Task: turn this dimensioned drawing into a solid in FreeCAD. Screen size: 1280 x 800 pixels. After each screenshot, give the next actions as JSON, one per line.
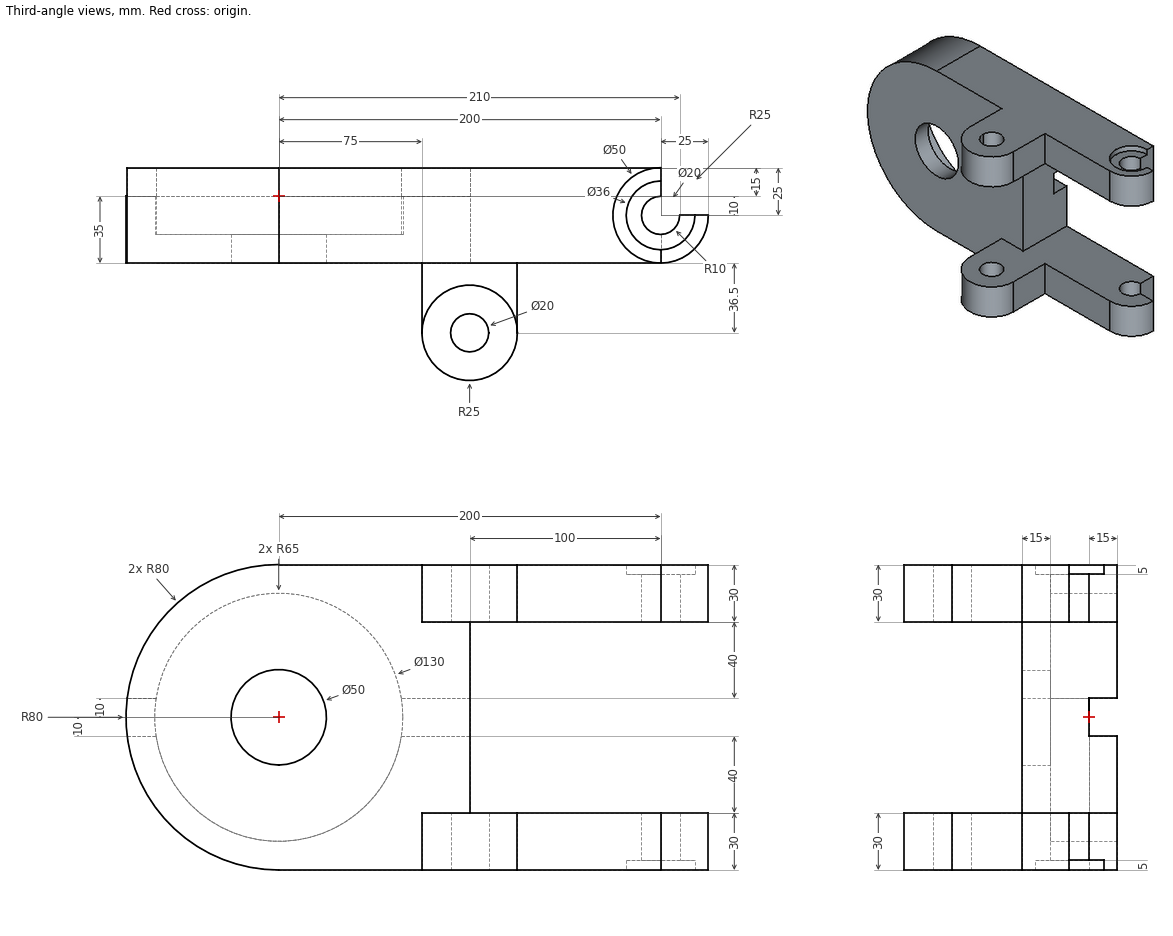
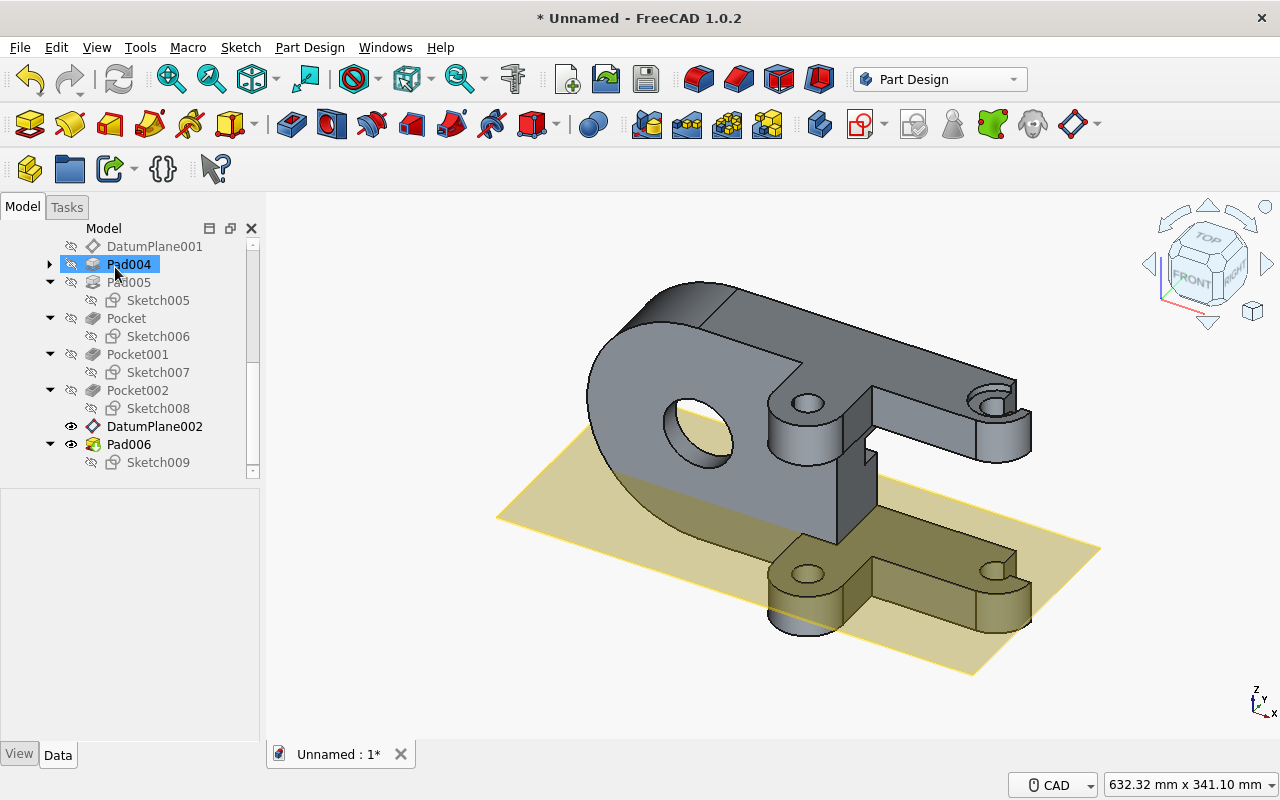
{"action": "left_click", "coordinate": [116, 426]}
{"action": "key", "text": "space"}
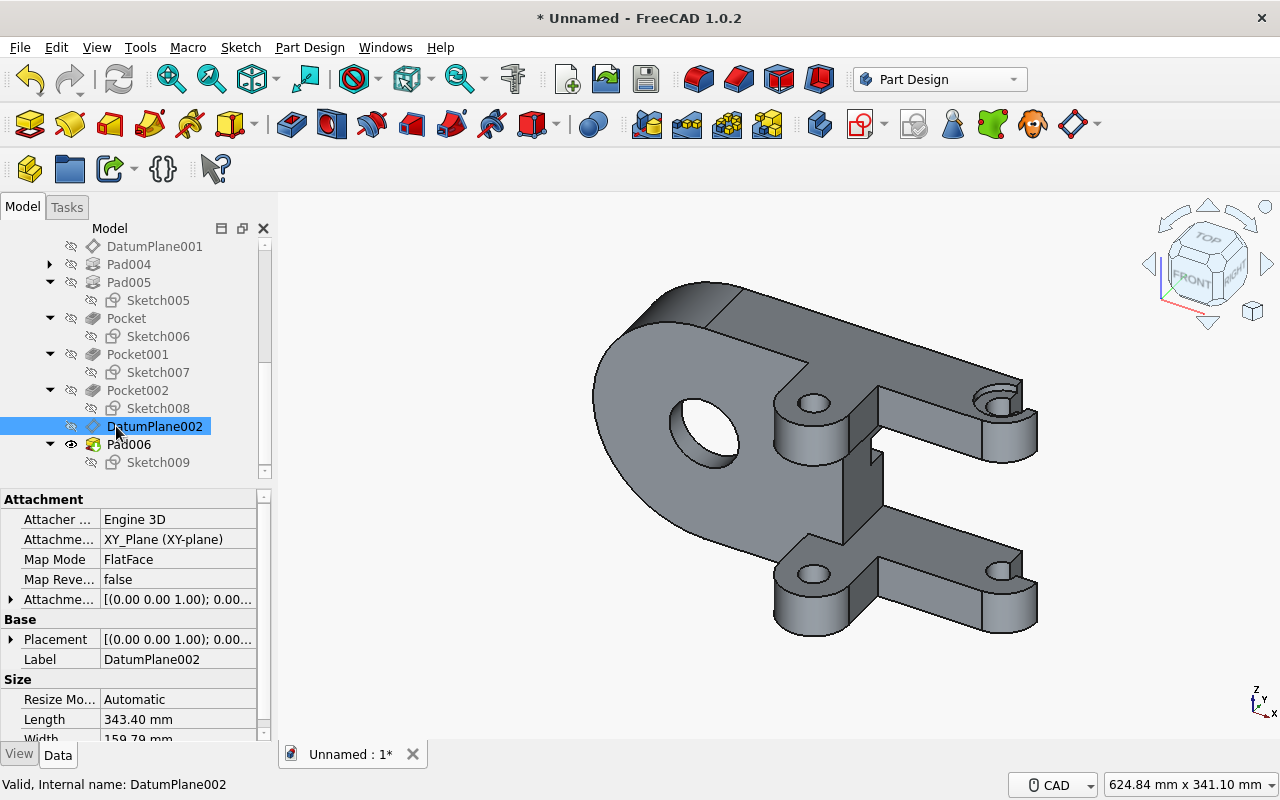
{"action": "scroll", "coordinate": [140, 350], "scroll_direction": "down", "scroll_amount": 3}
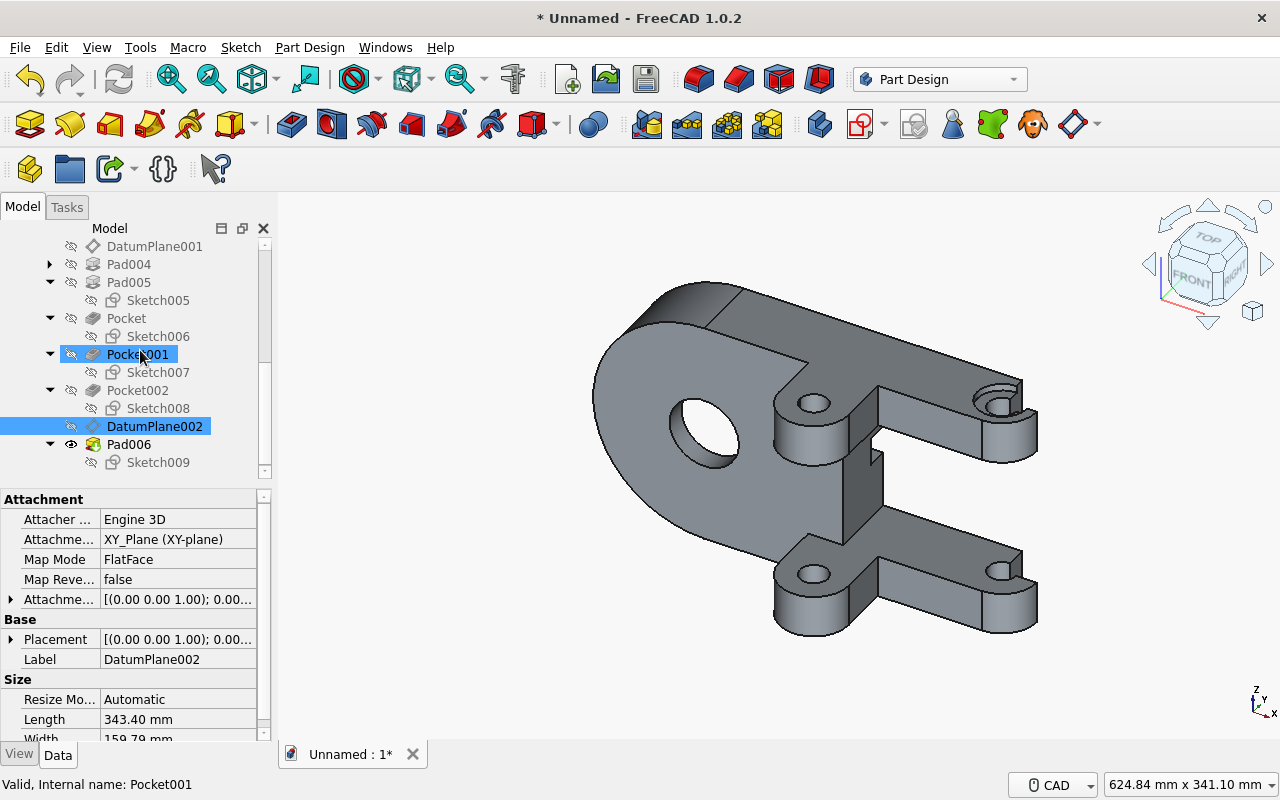
{"action": "scroll", "coordinate": [140, 350], "scroll_direction": "up", "scroll_amount": 15}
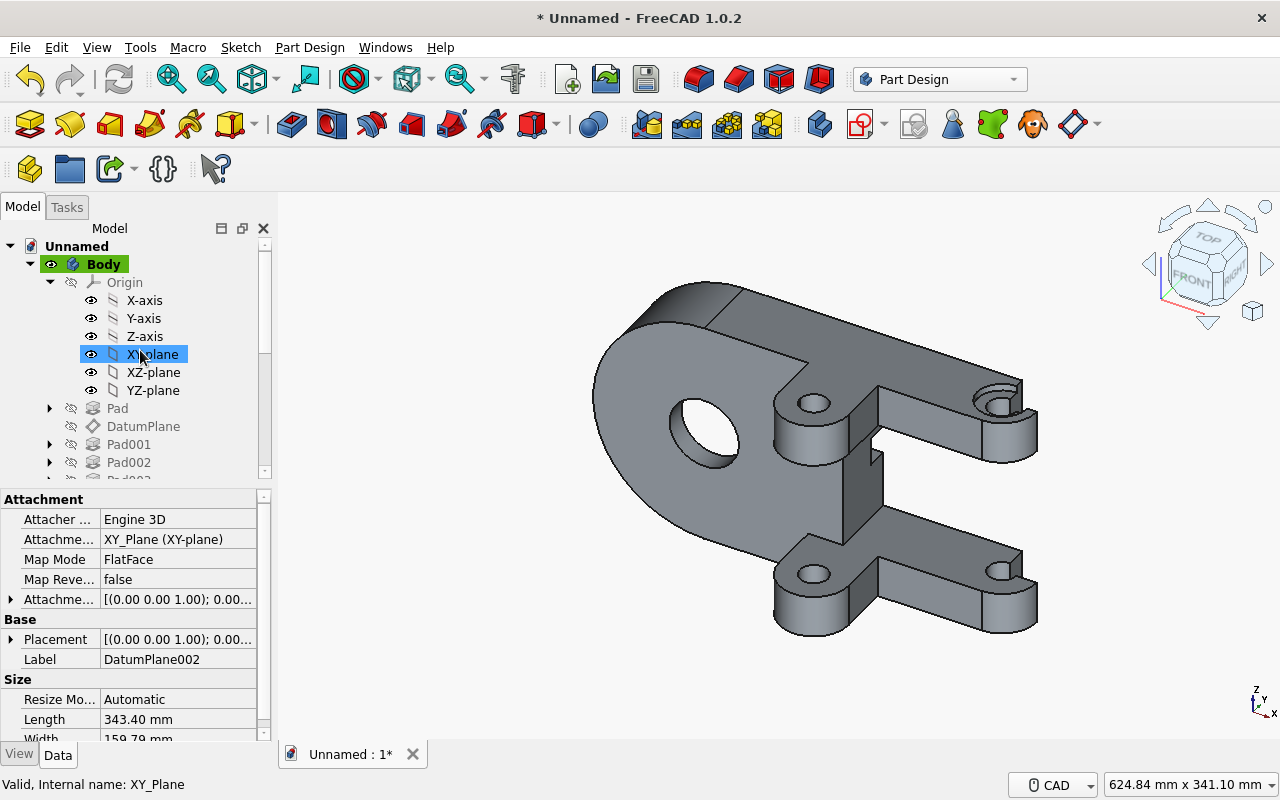
{"action": "left_click", "coordinate": [136, 354]}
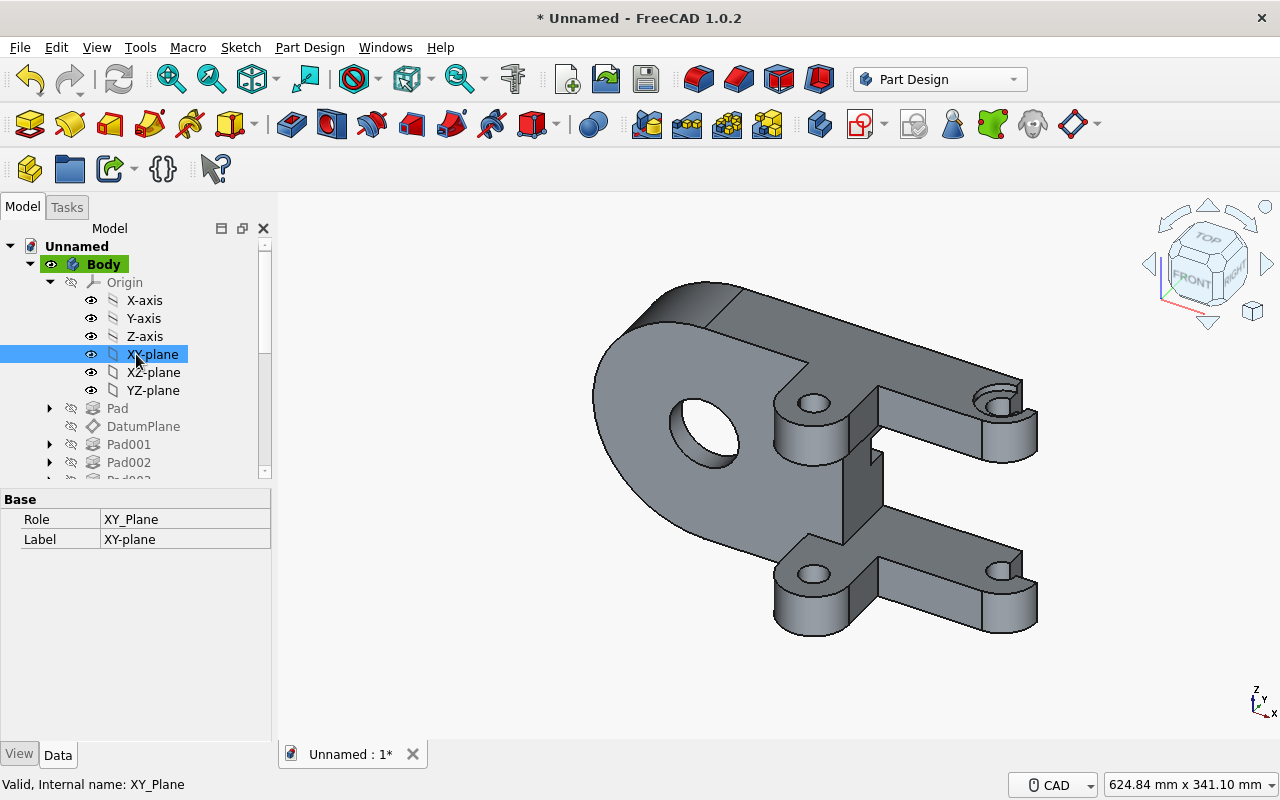
{"action": "left_click", "coordinate": [1074, 124]}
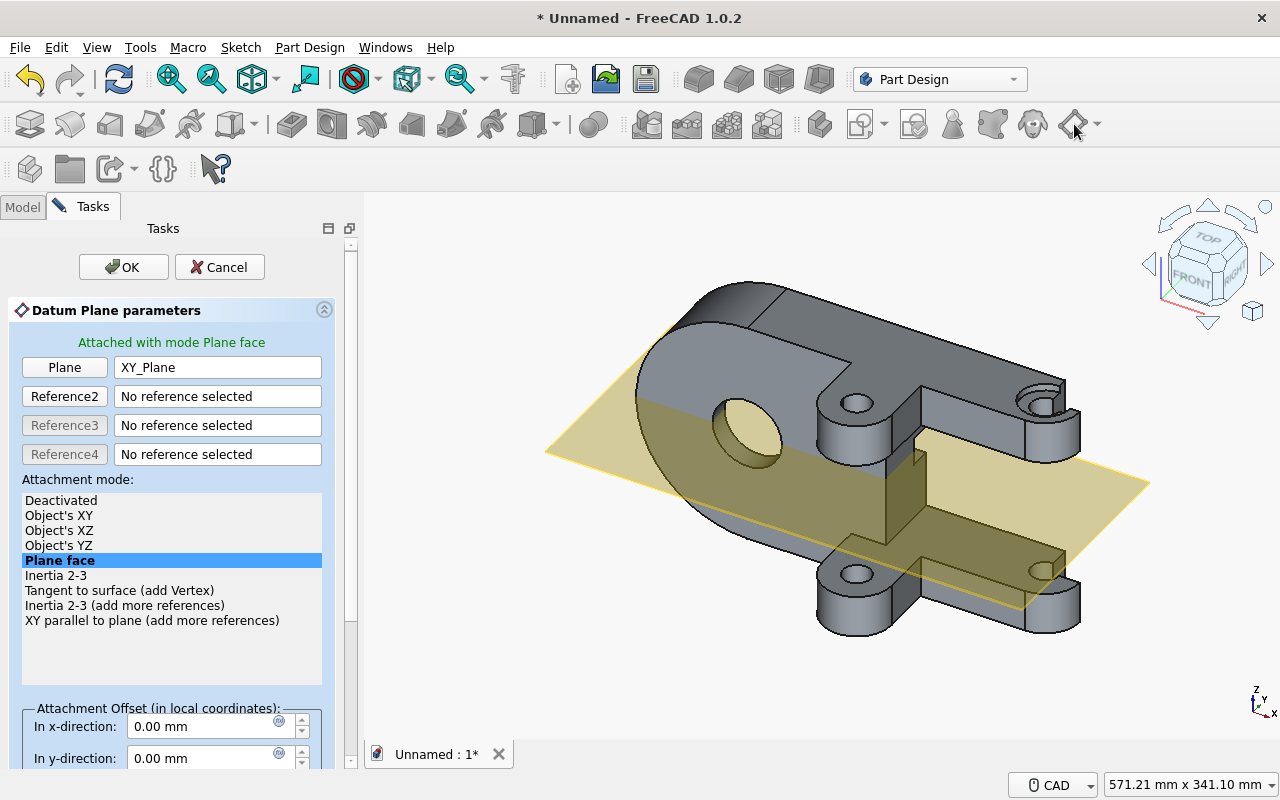
{"action": "scroll", "coordinate": [351, 503], "scroll_direction": "down", "scroll_amount": 2}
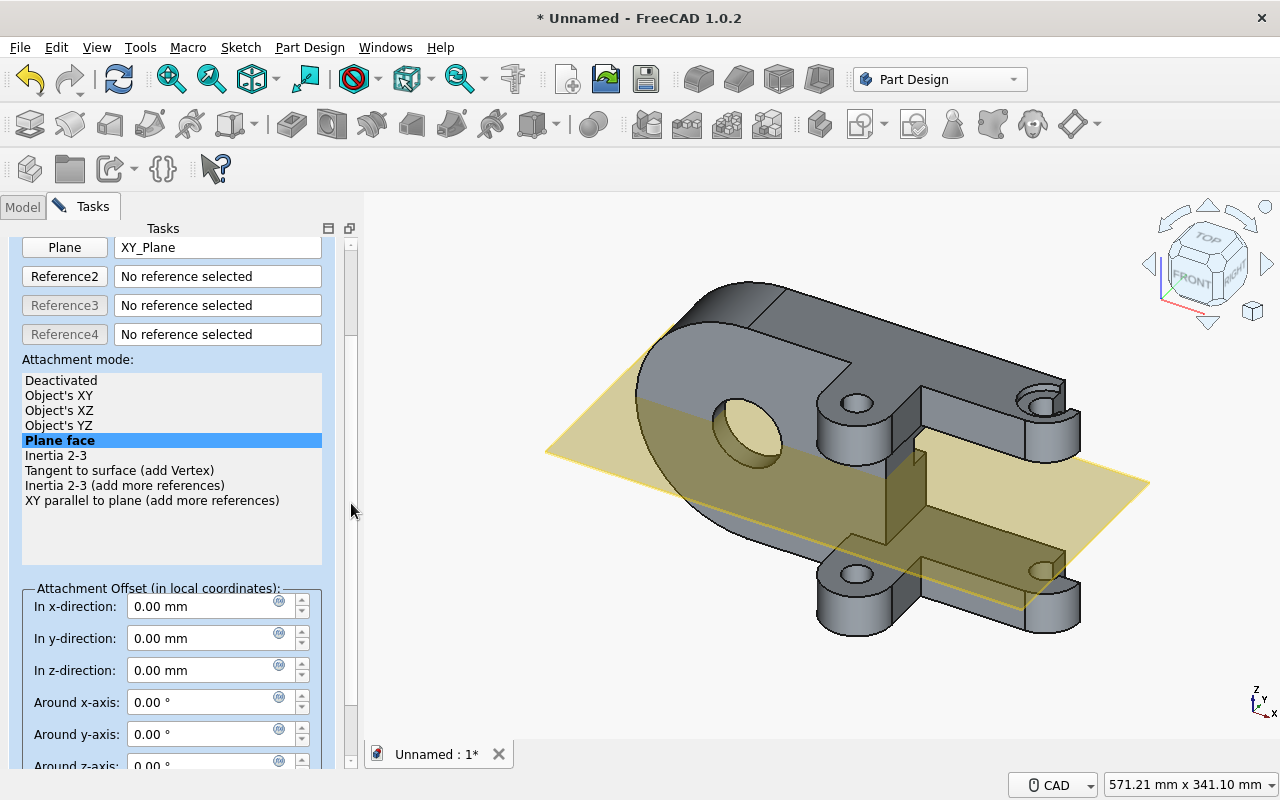
{"action": "triple_click", "coordinate": [210, 670]}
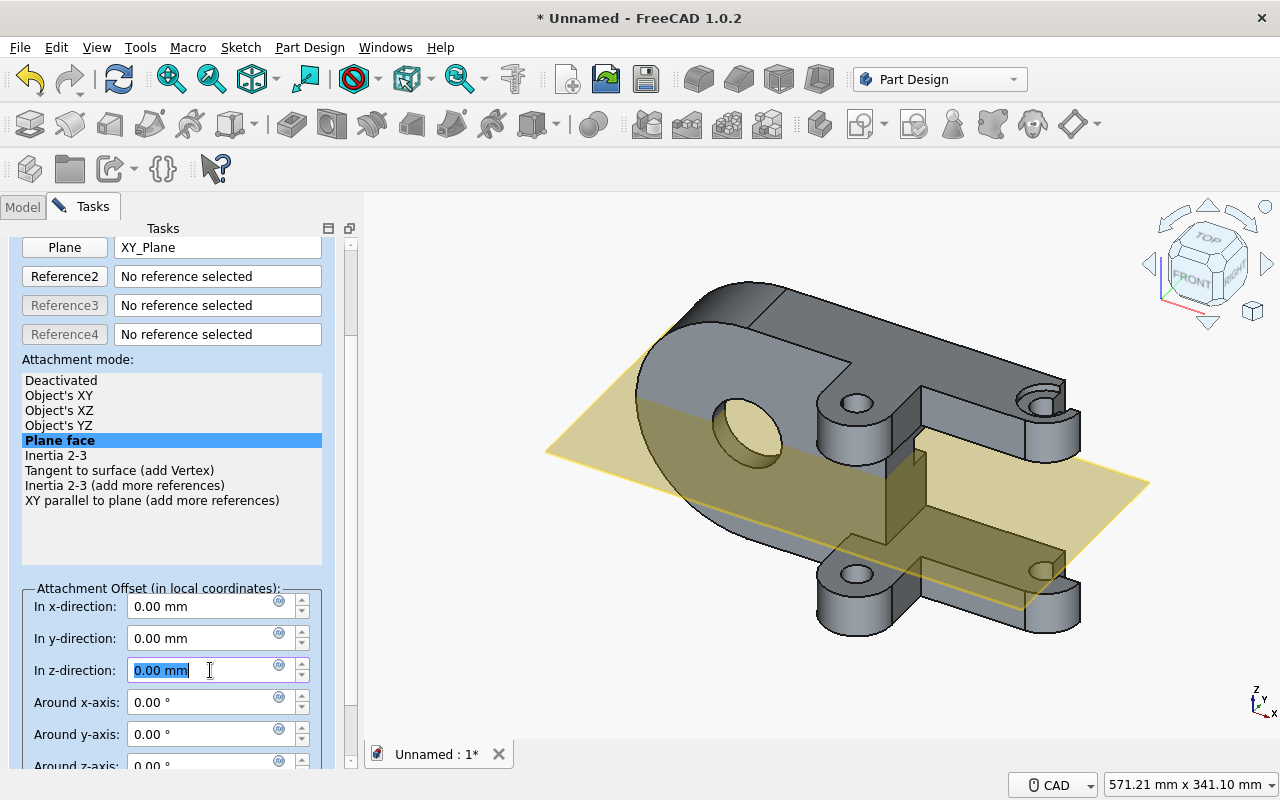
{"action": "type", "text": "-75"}
{"action": "key", "text": "Tab"}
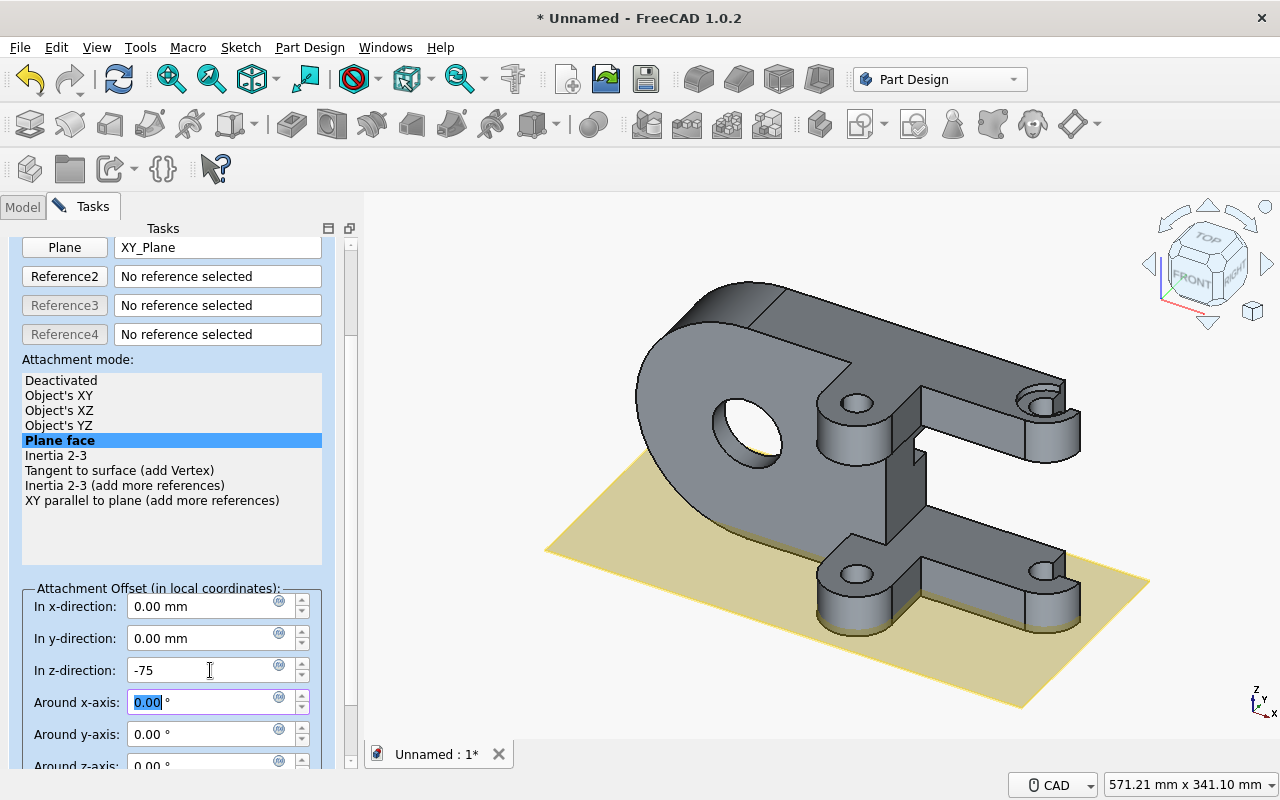
{"action": "scroll", "coordinate": [351, 503], "scroll_direction": "up", "scroll_amount": 3}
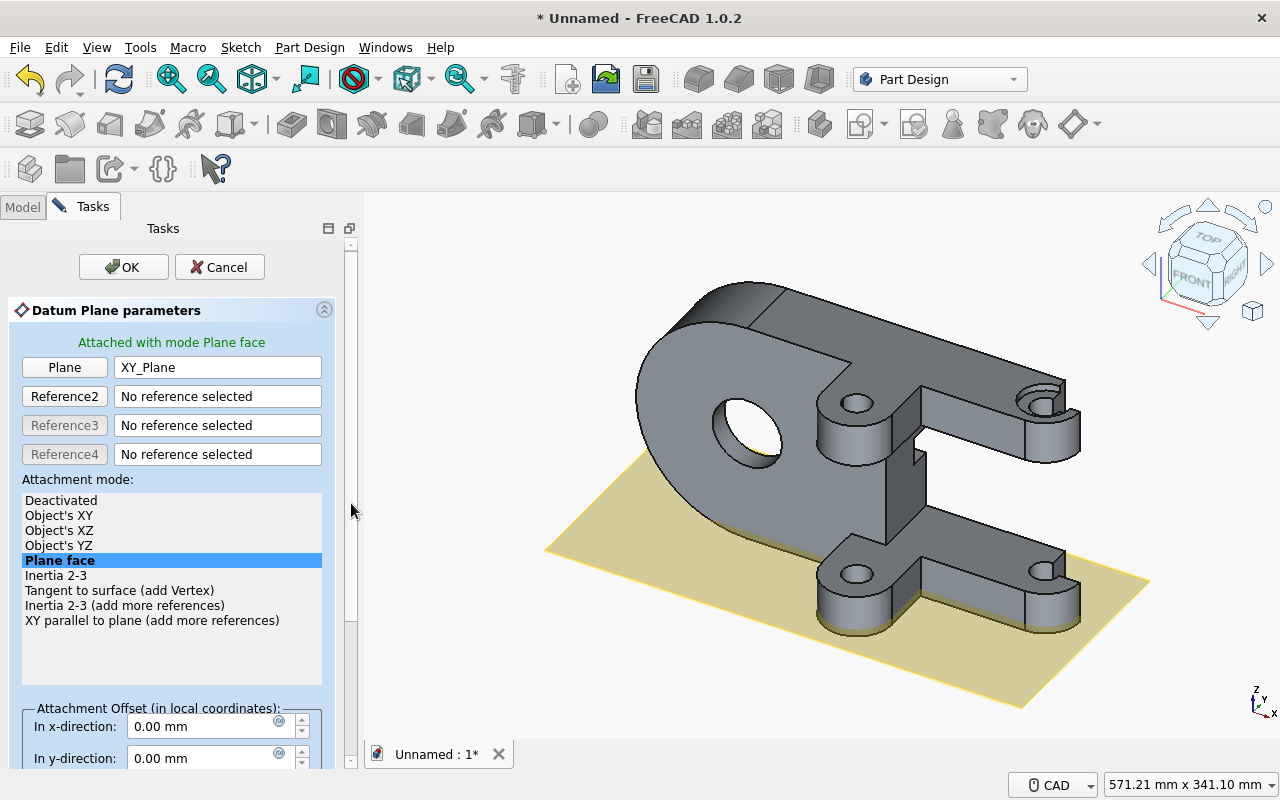
{"action": "left_click", "coordinate": [124, 267]}